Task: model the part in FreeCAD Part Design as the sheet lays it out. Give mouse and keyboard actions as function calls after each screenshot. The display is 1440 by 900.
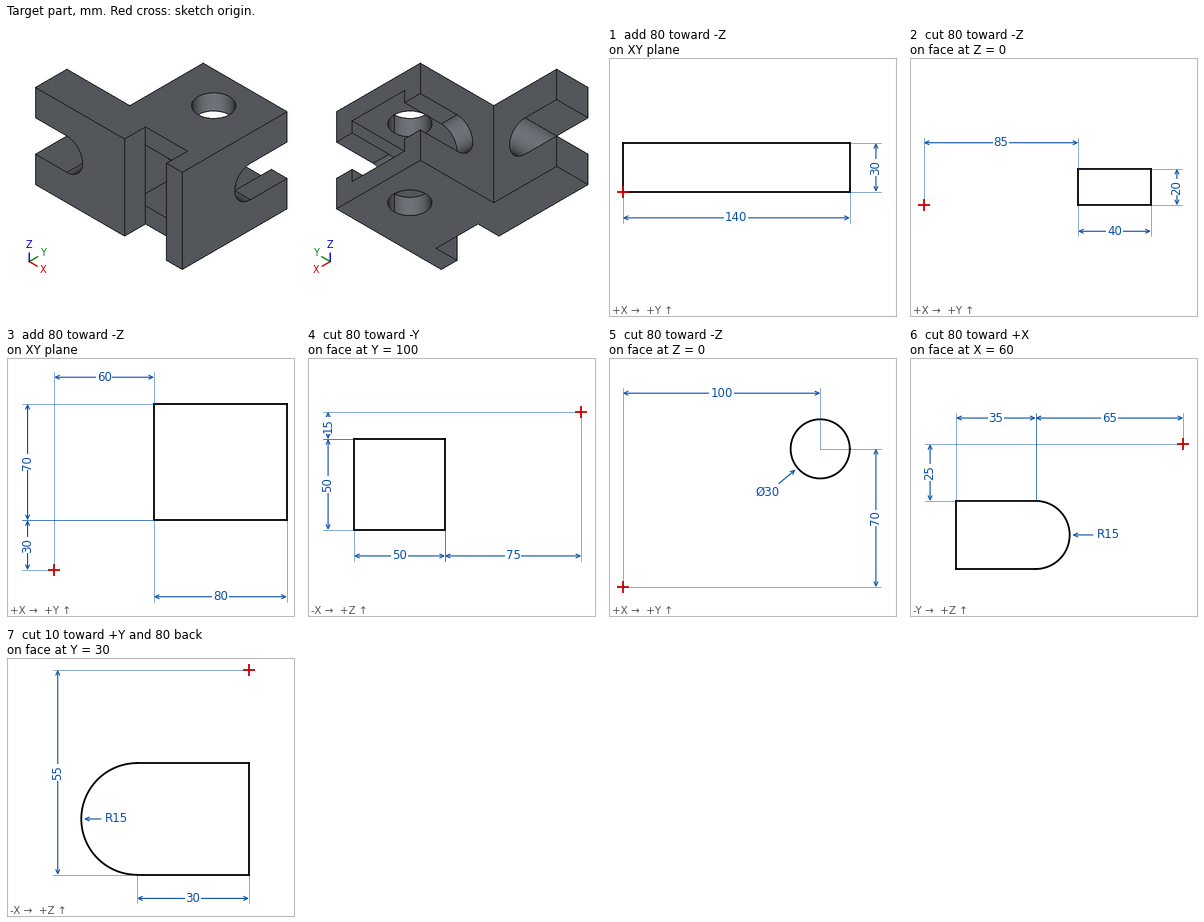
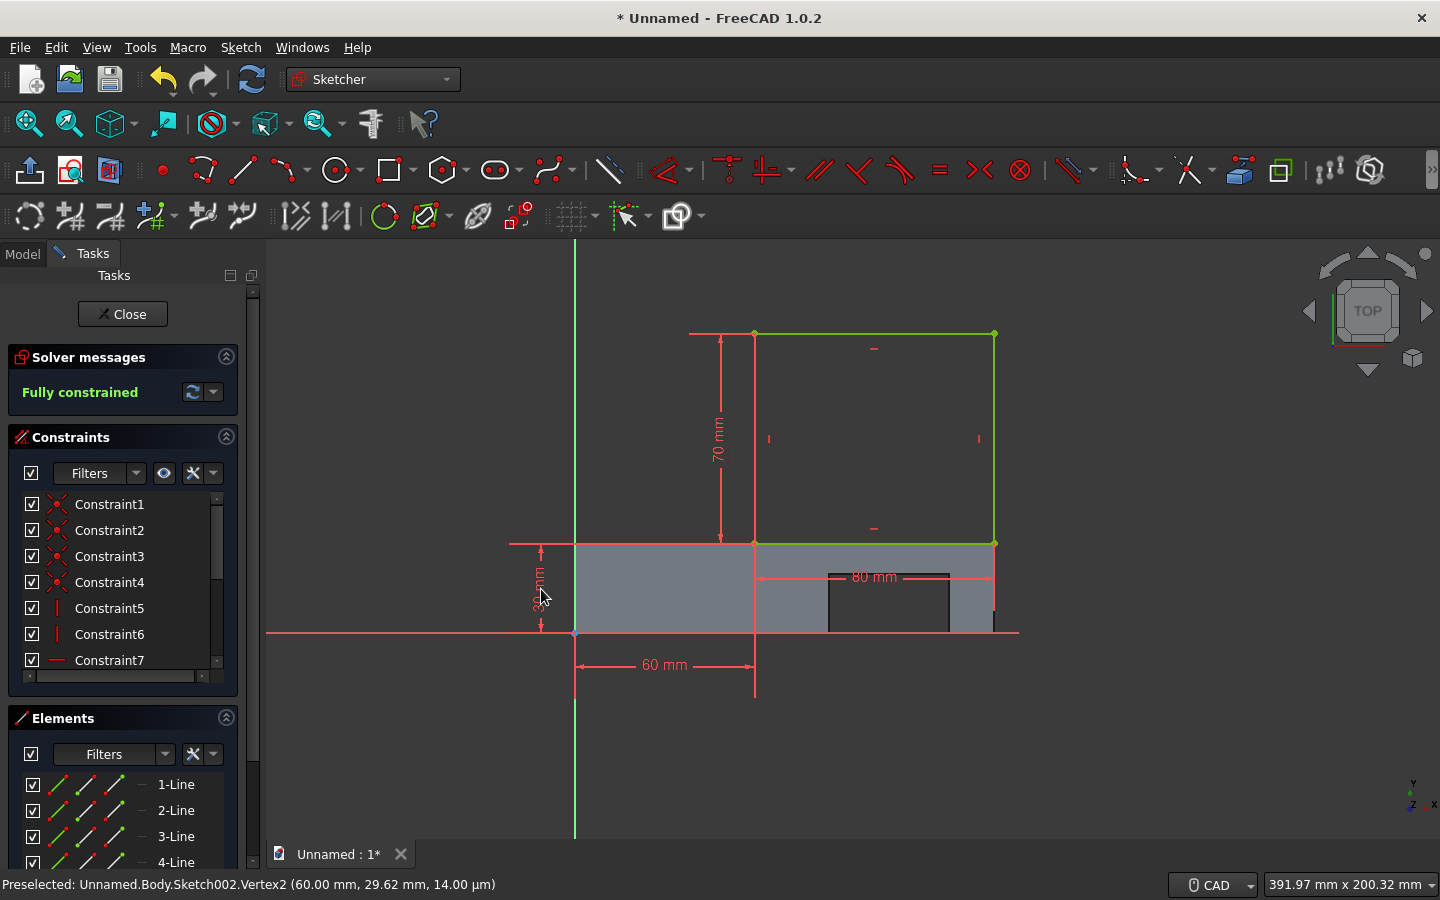
click(123, 314)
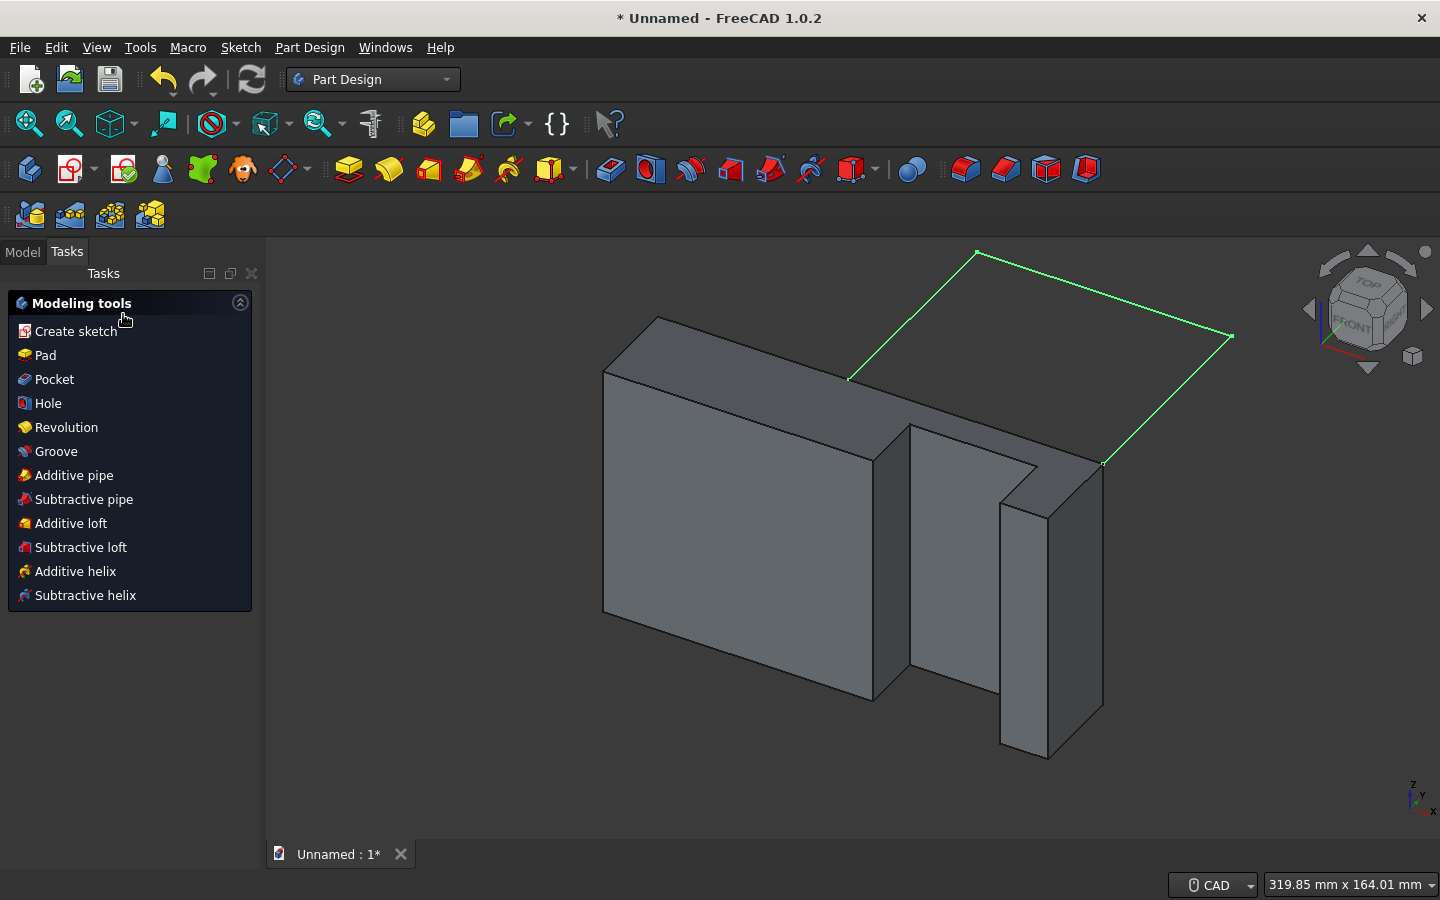
click(350, 170)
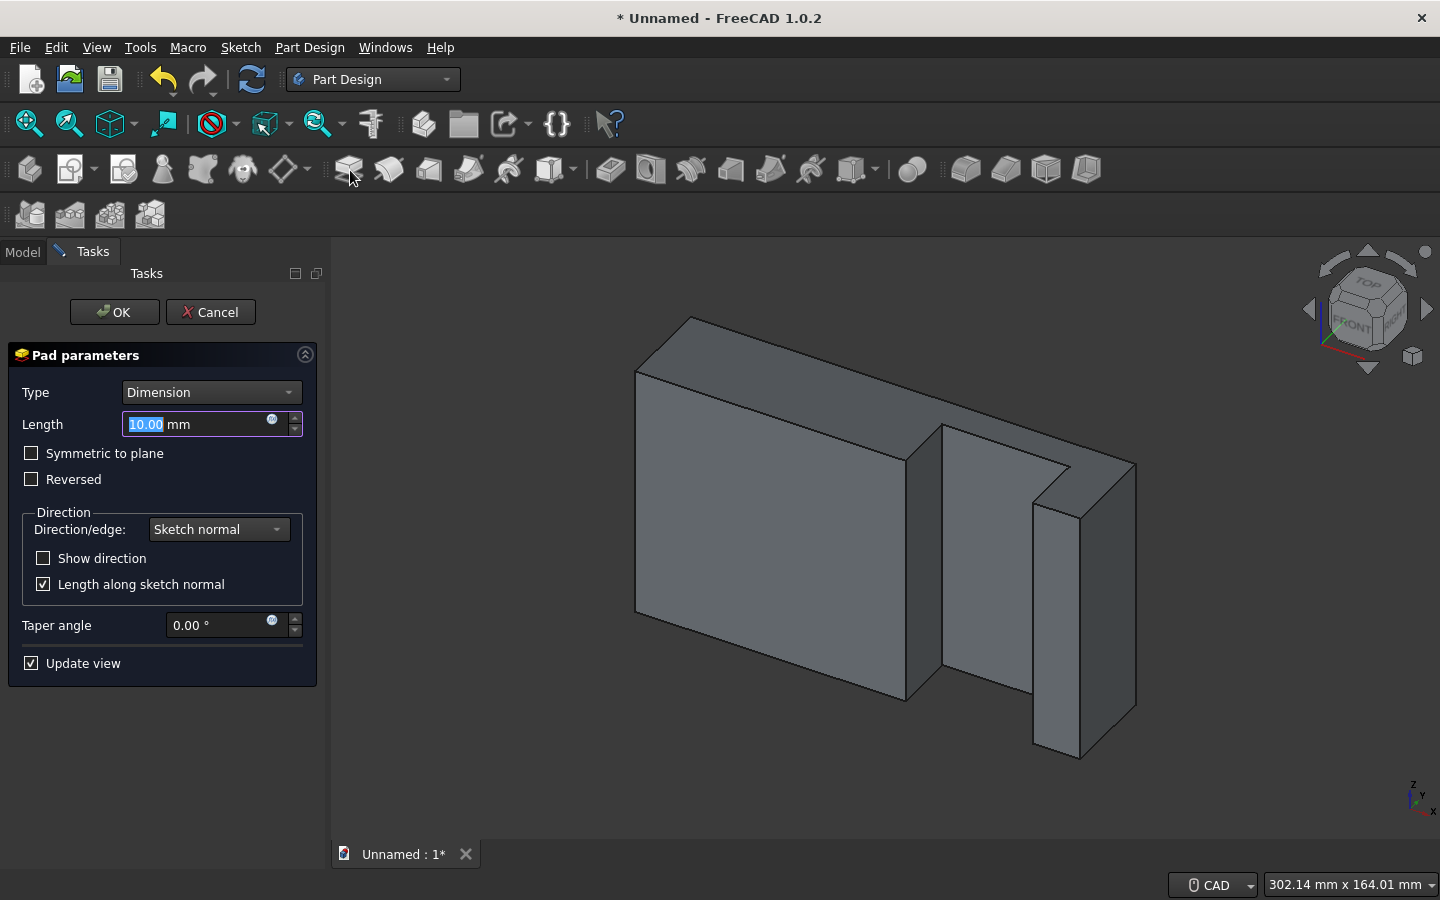
text(80)
key(Tab)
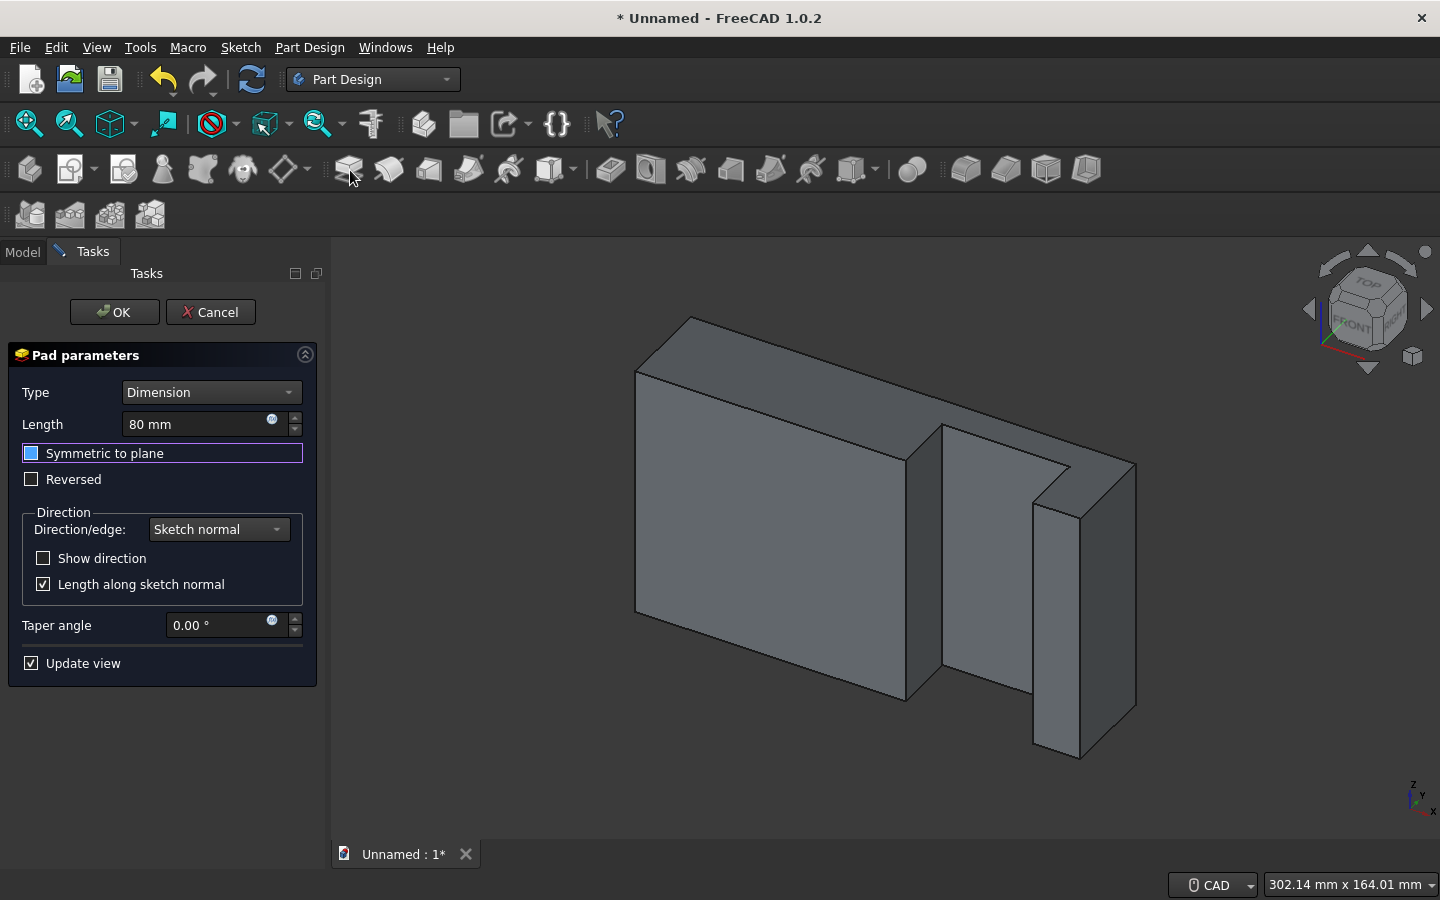
click(30, 479)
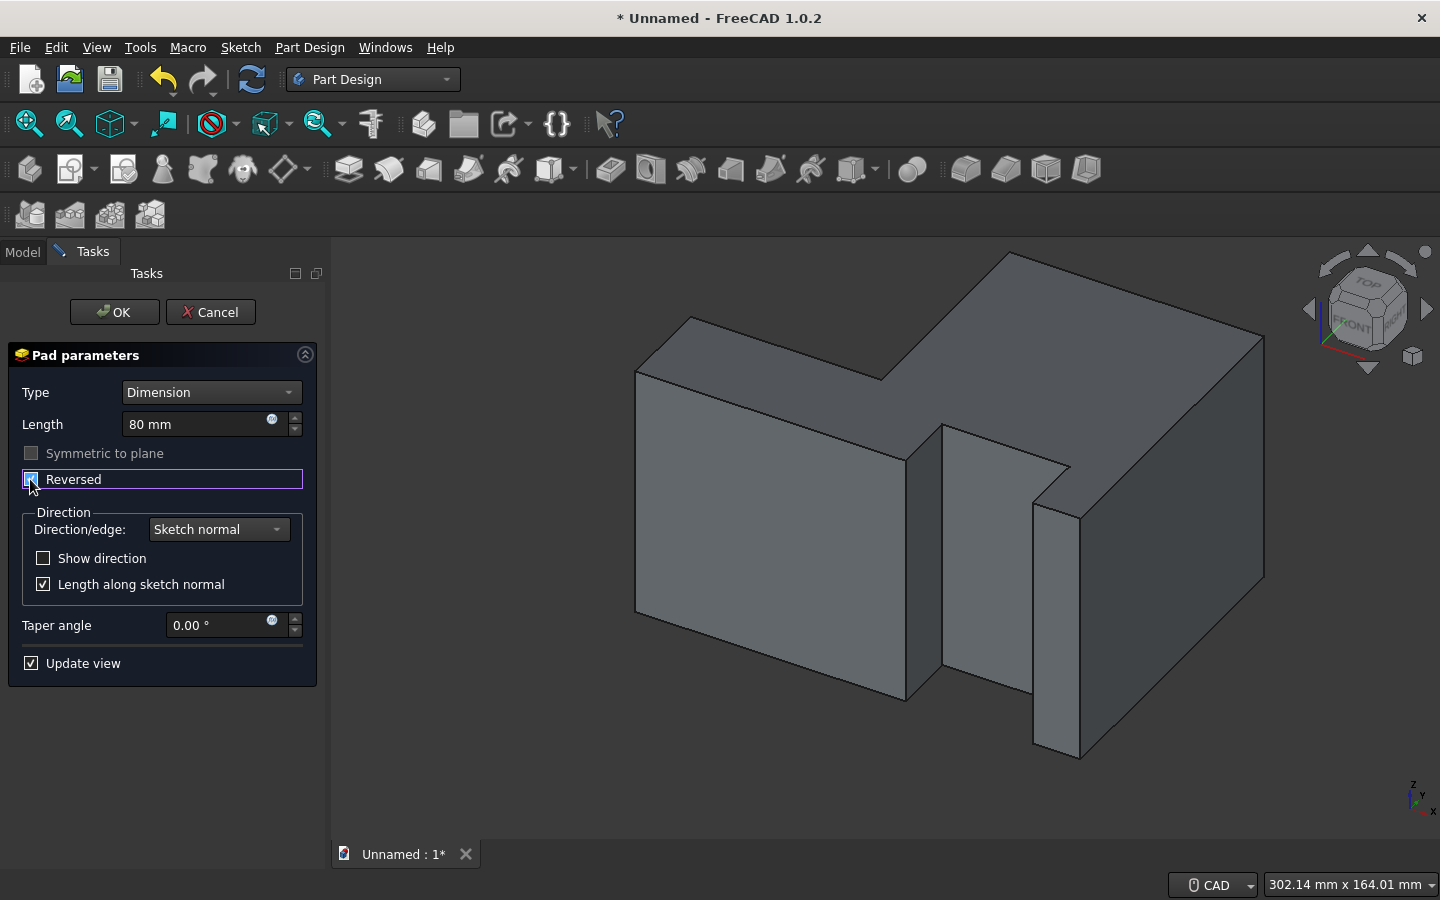
click(115, 312)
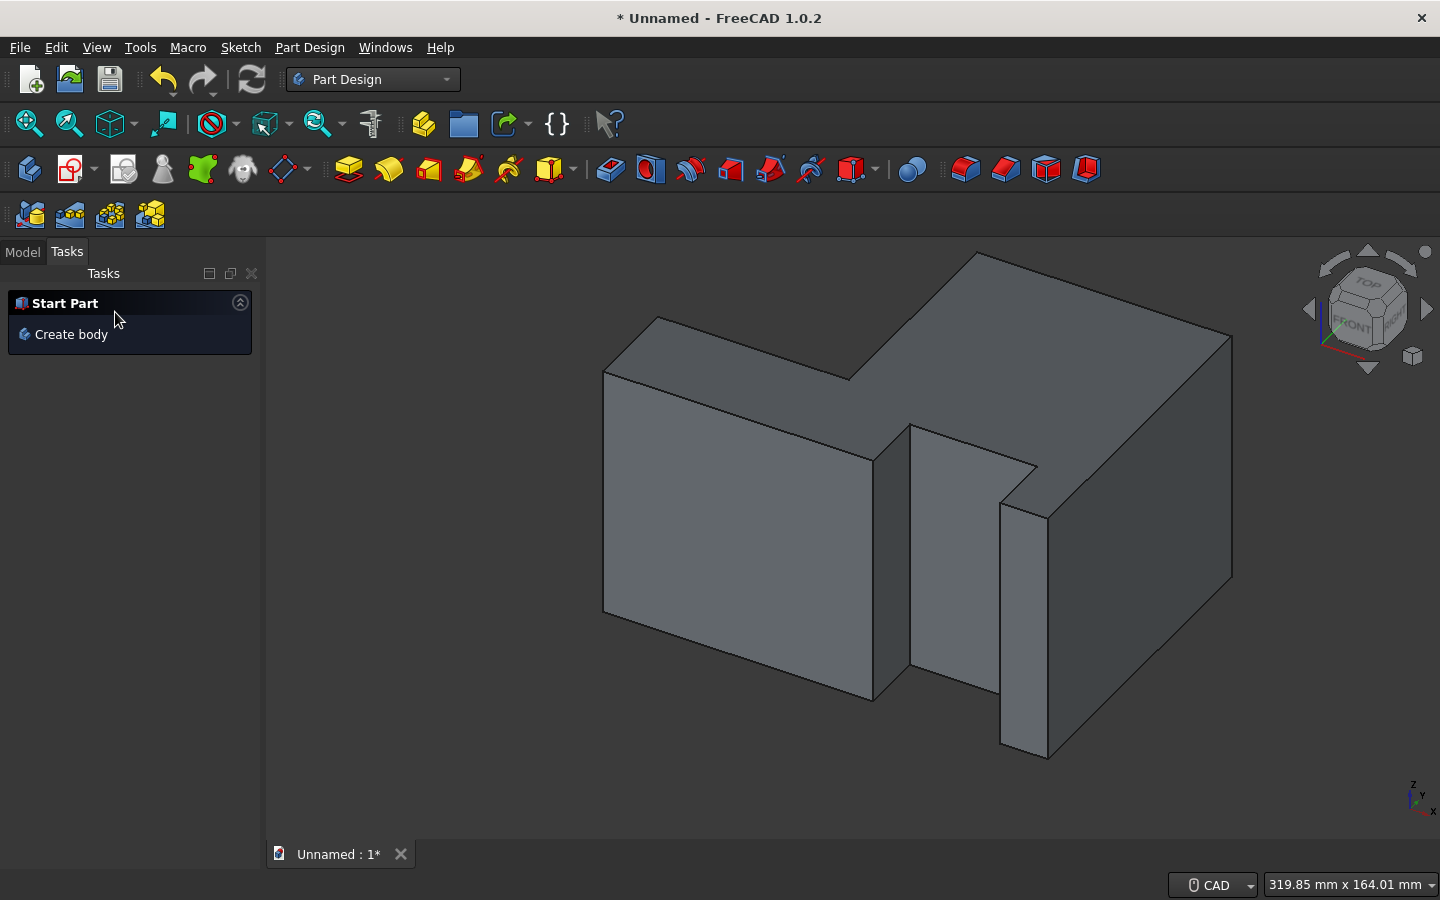
key(v)
key(f)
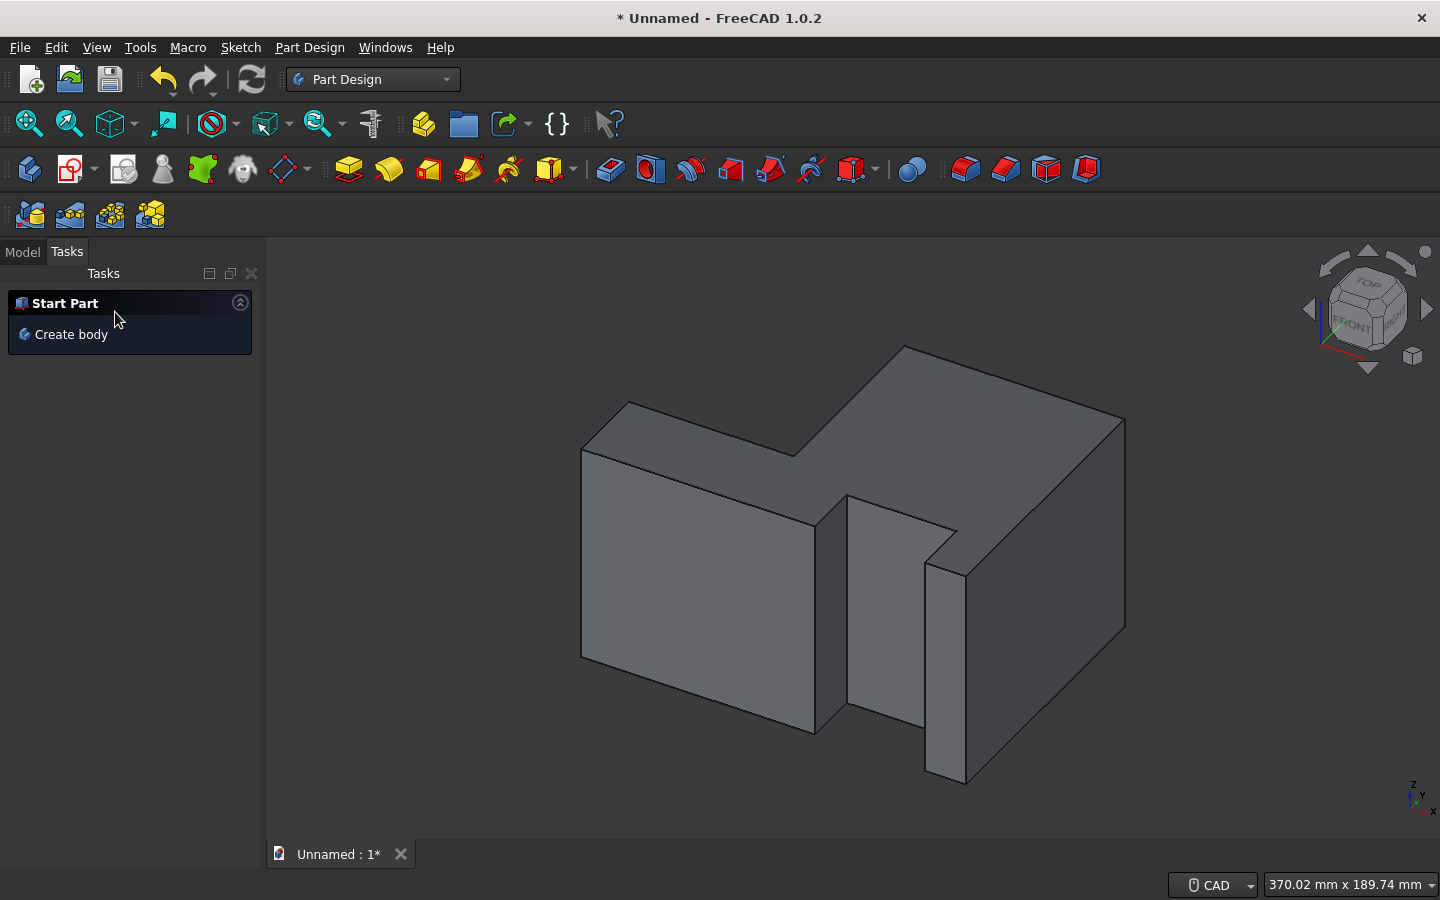
key(4)